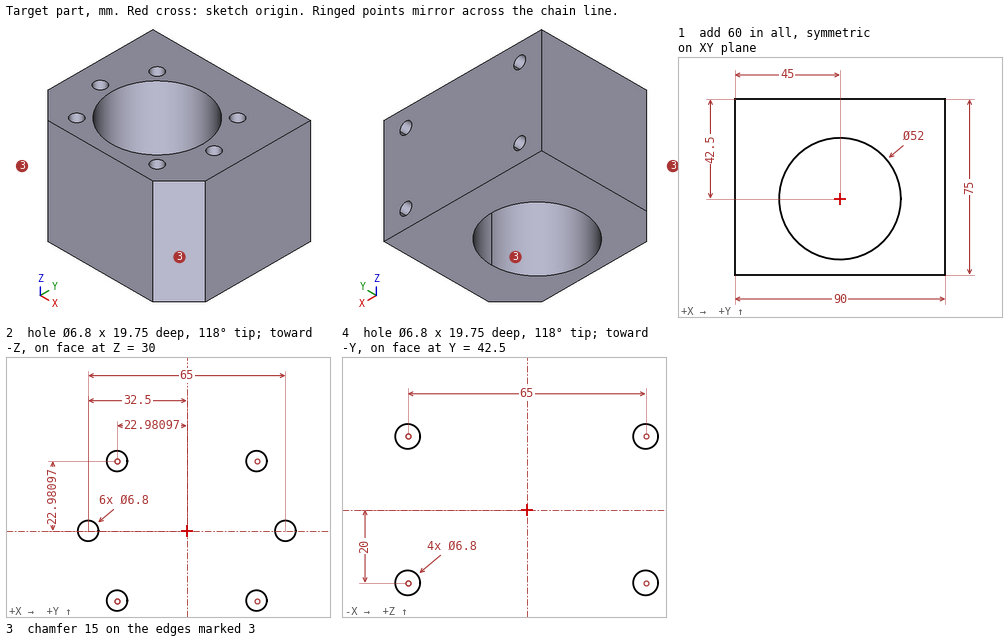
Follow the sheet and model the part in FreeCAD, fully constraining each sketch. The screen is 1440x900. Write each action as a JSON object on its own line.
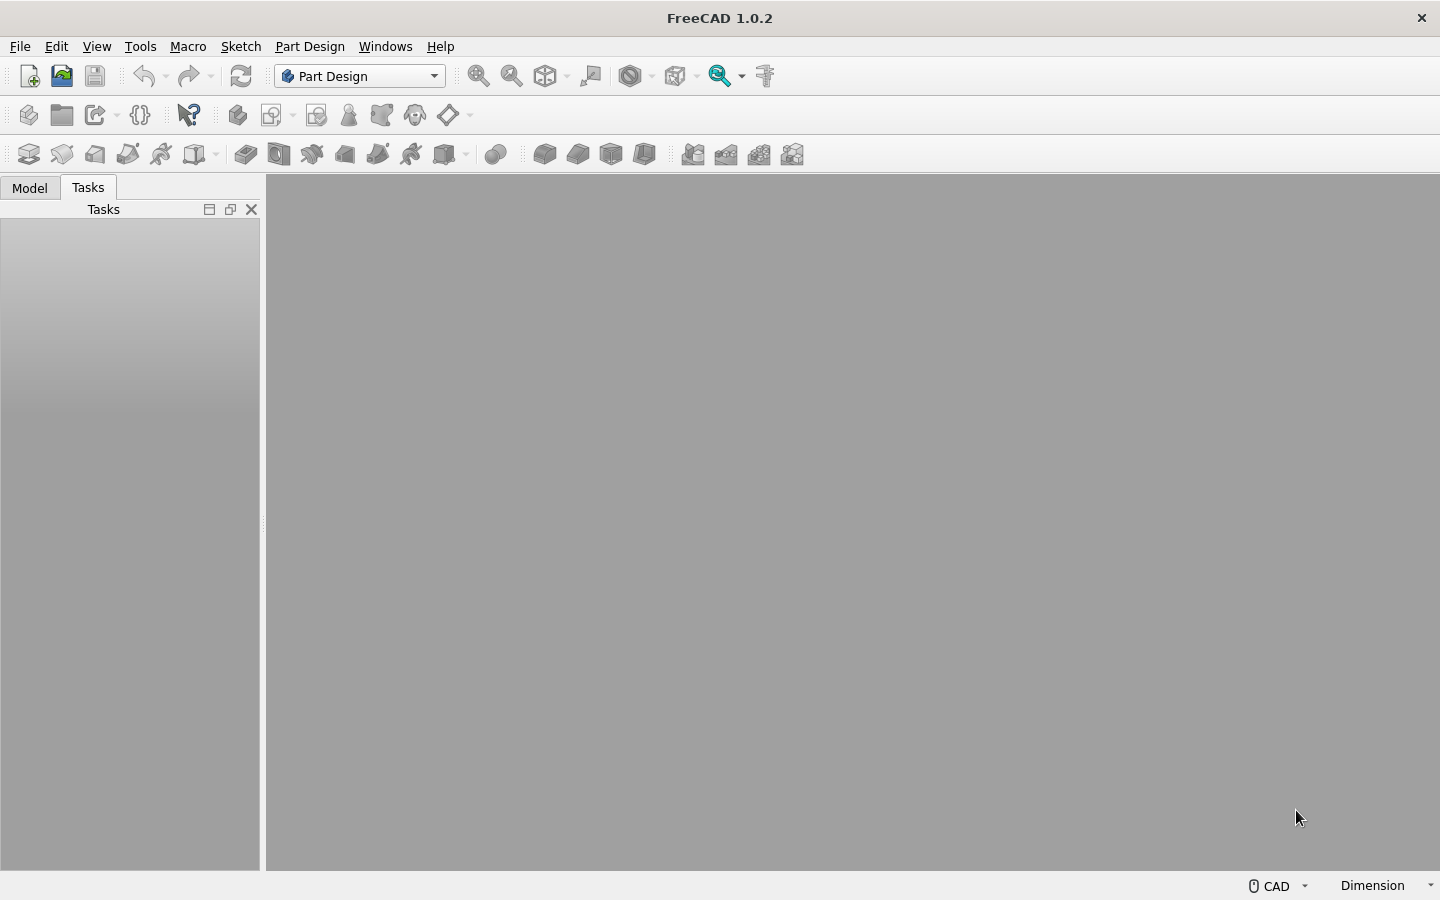
{"action": "left_click", "coordinate": [29, 76]}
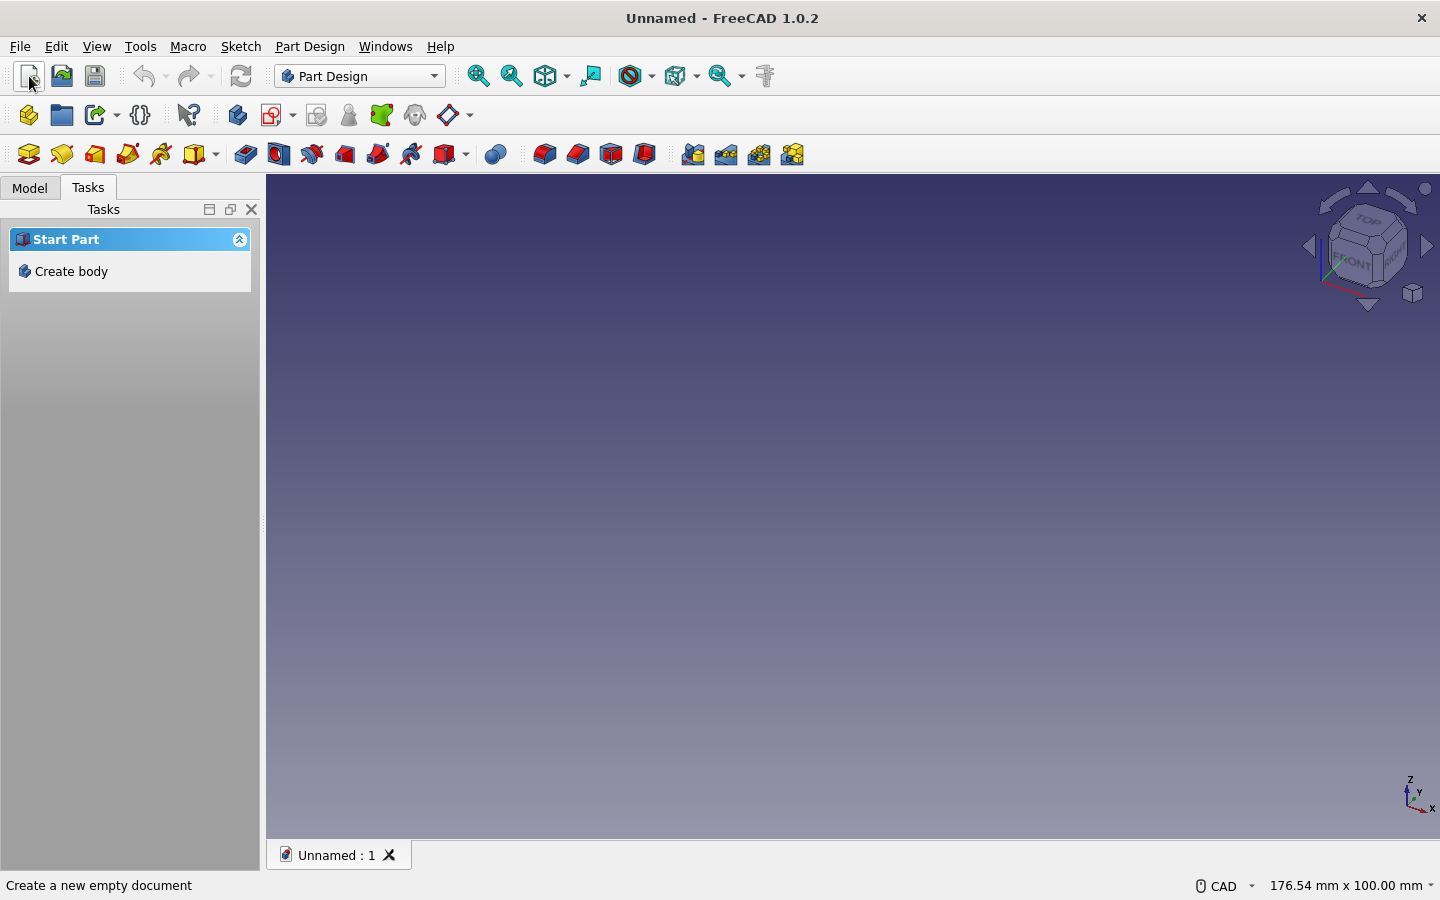
{"action": "left_click", "coordinate": [270, 116]}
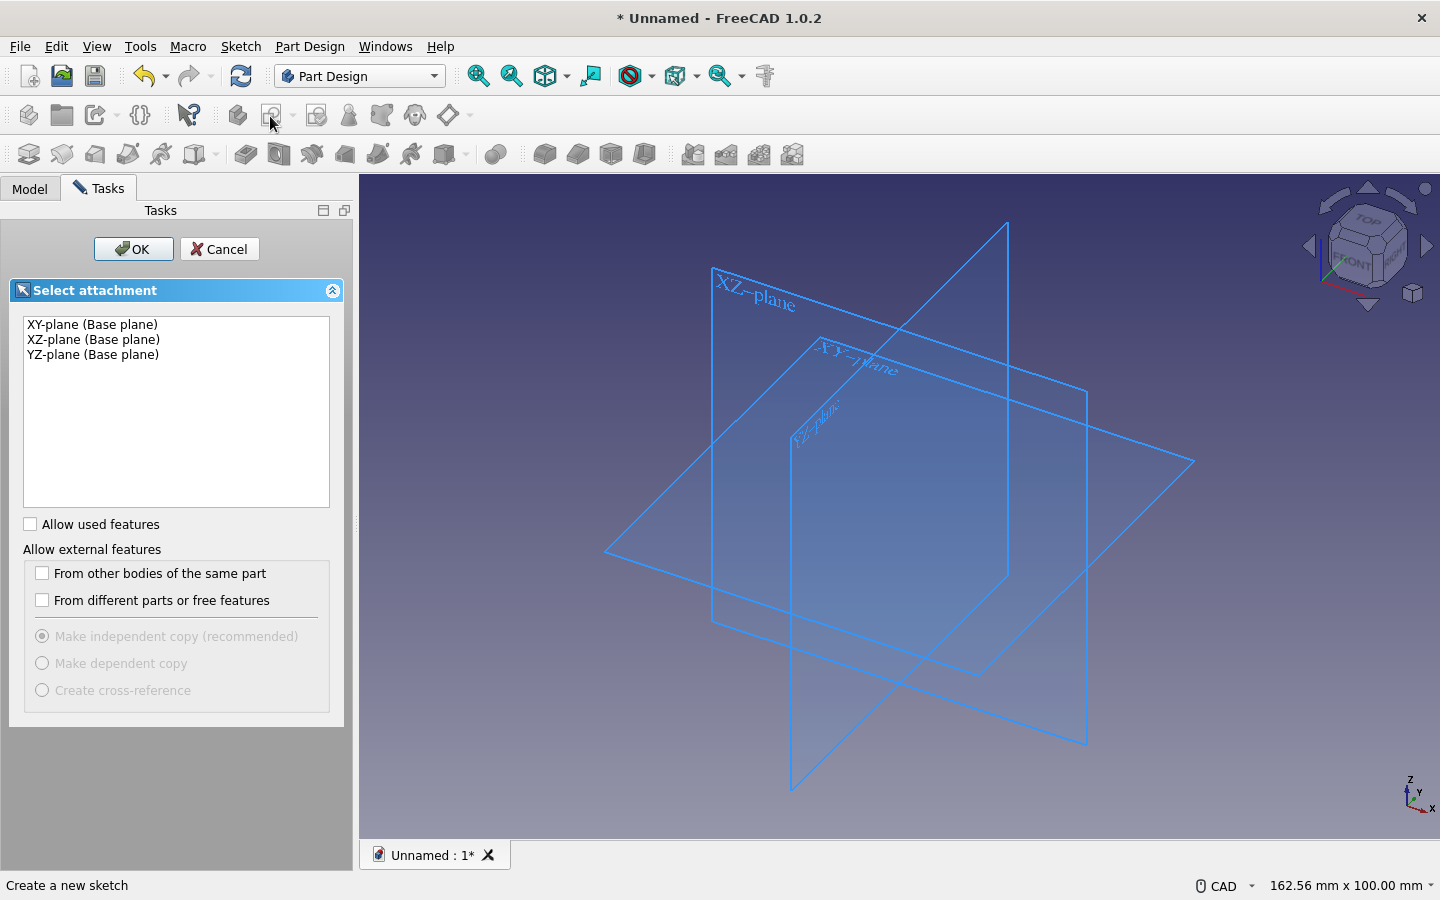
{"action": "left_click", "coordinate": [84, 324]}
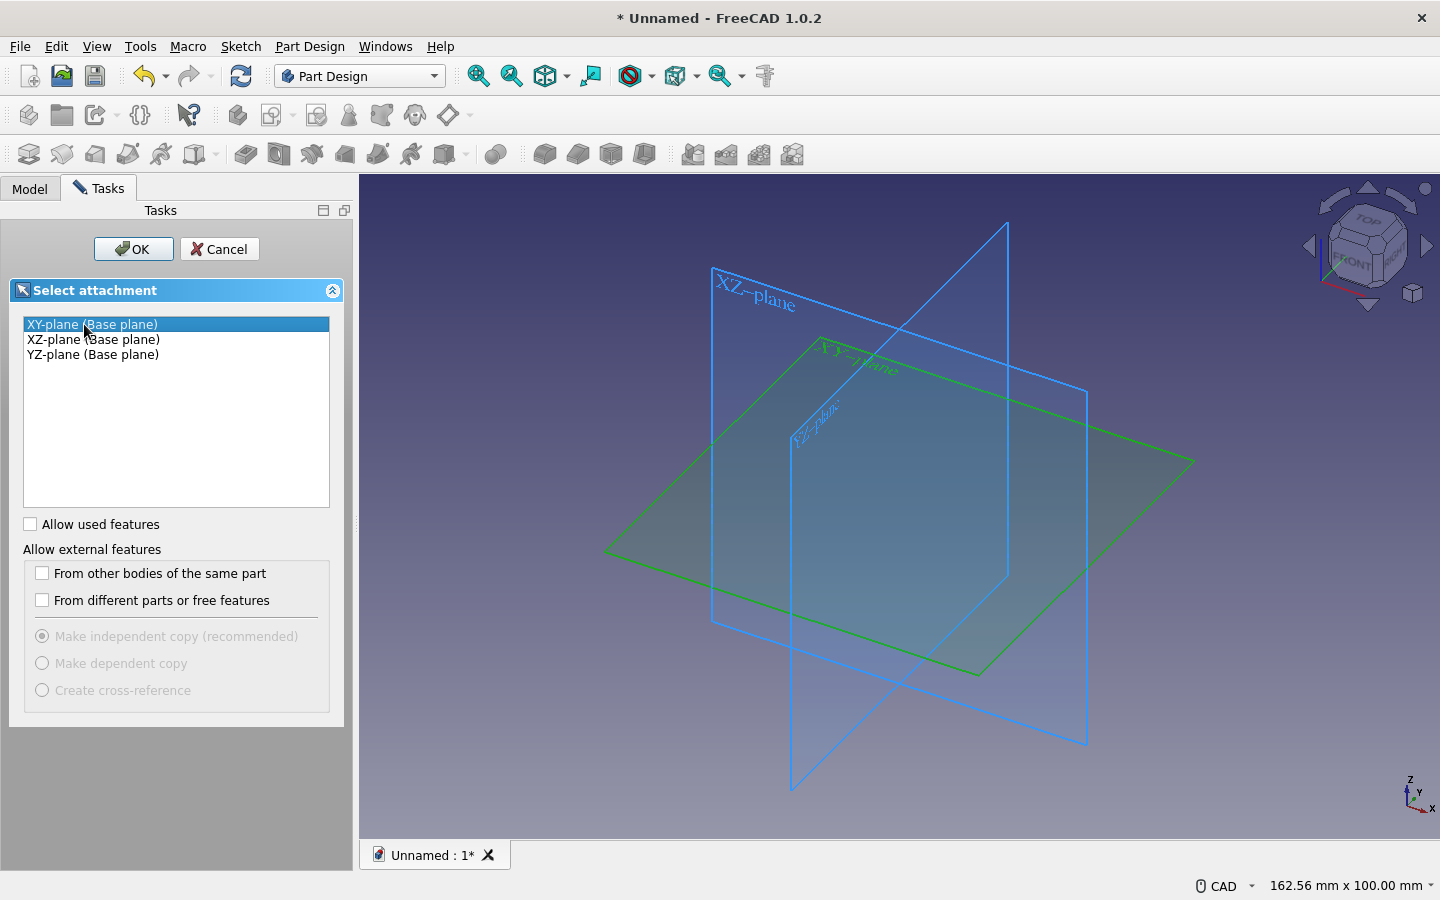
{"action": "left_click", "coordinate": [134, 249]}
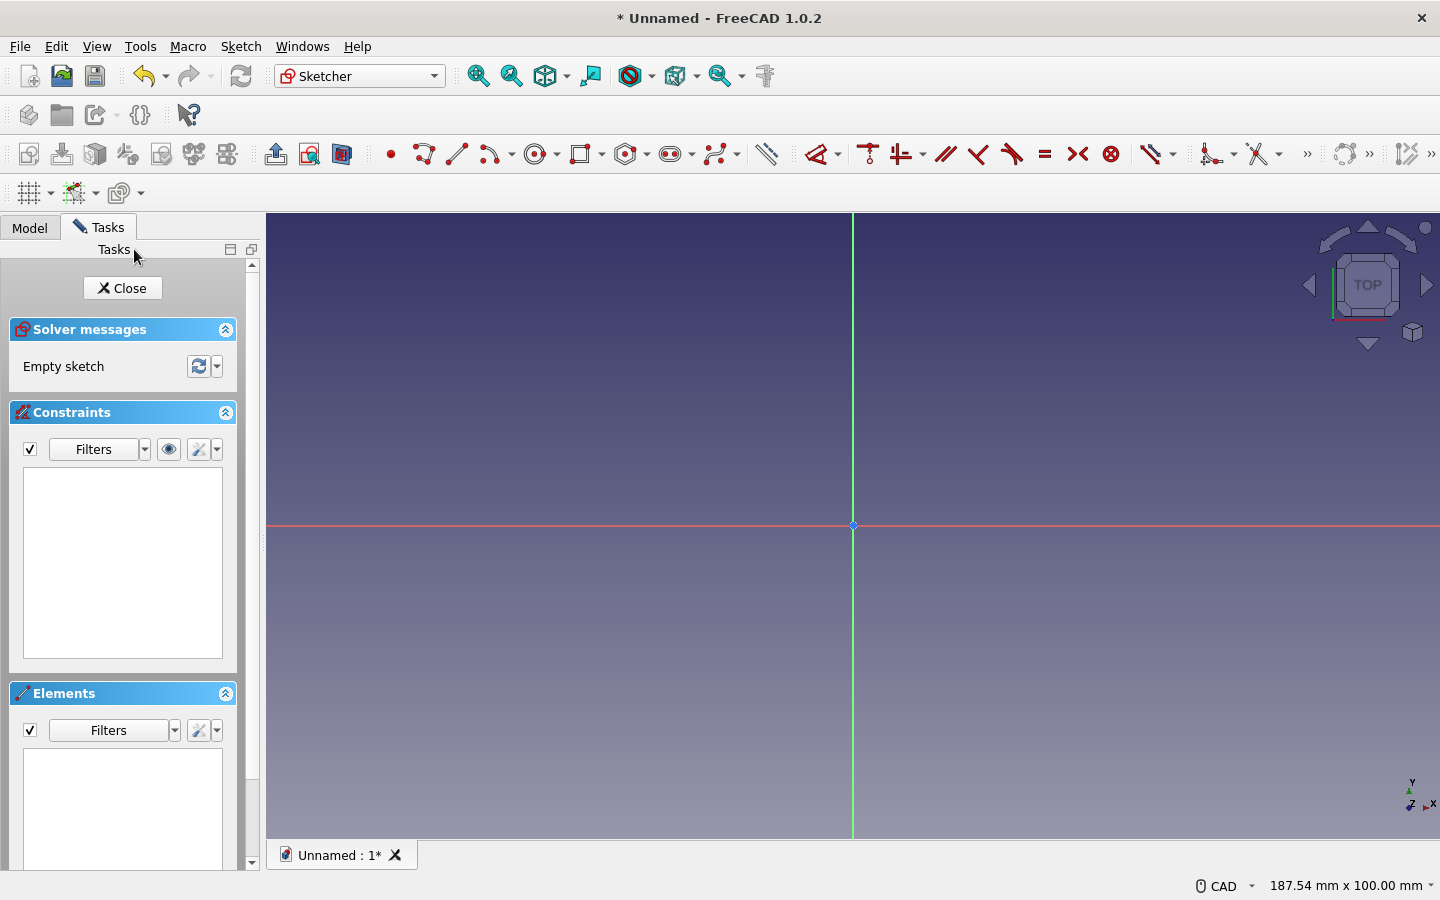
{"action": "scroll", "coordinate": [475, 667], "scroll_direction": "down", "scroll_amount": 1}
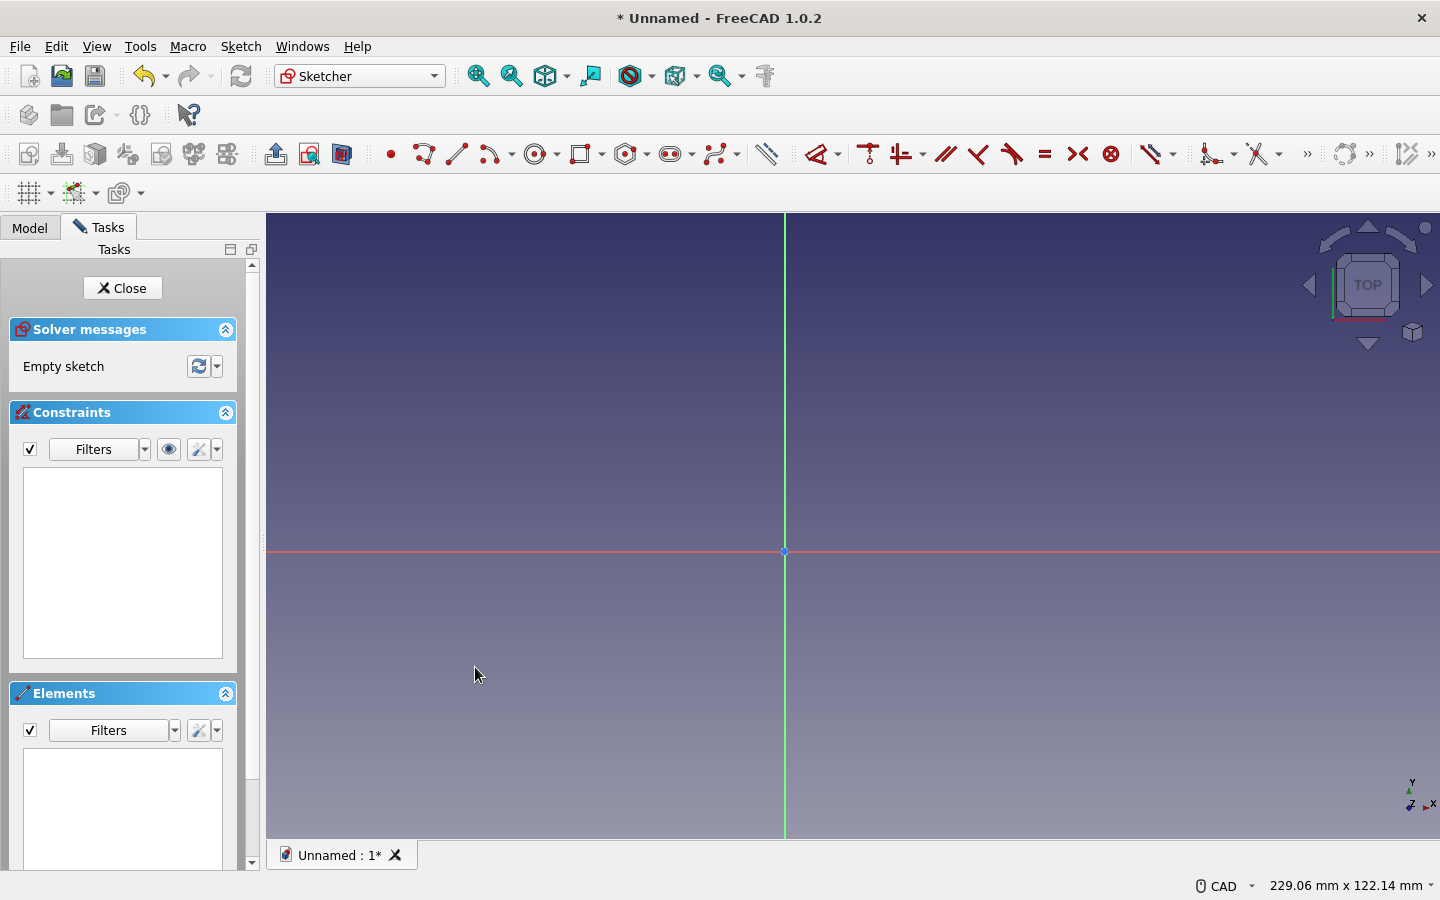
{"action": "left_click", "coordinate": [580, 154]}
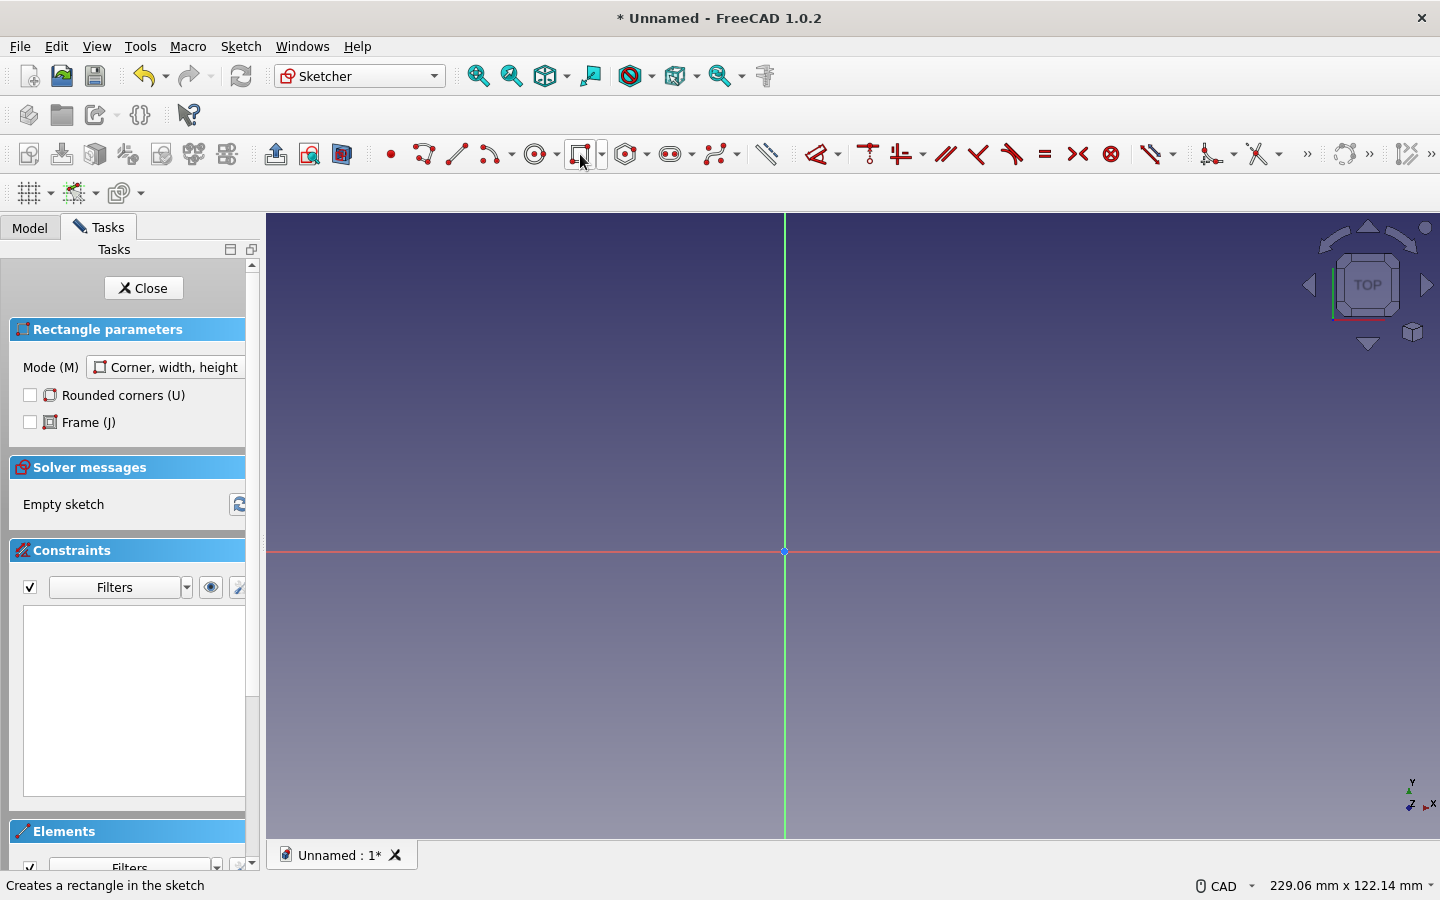
{"action": "left_click", "coordinate": [554, 334]}
{"action": "mouse_move", "coordinate": [1015, 718]}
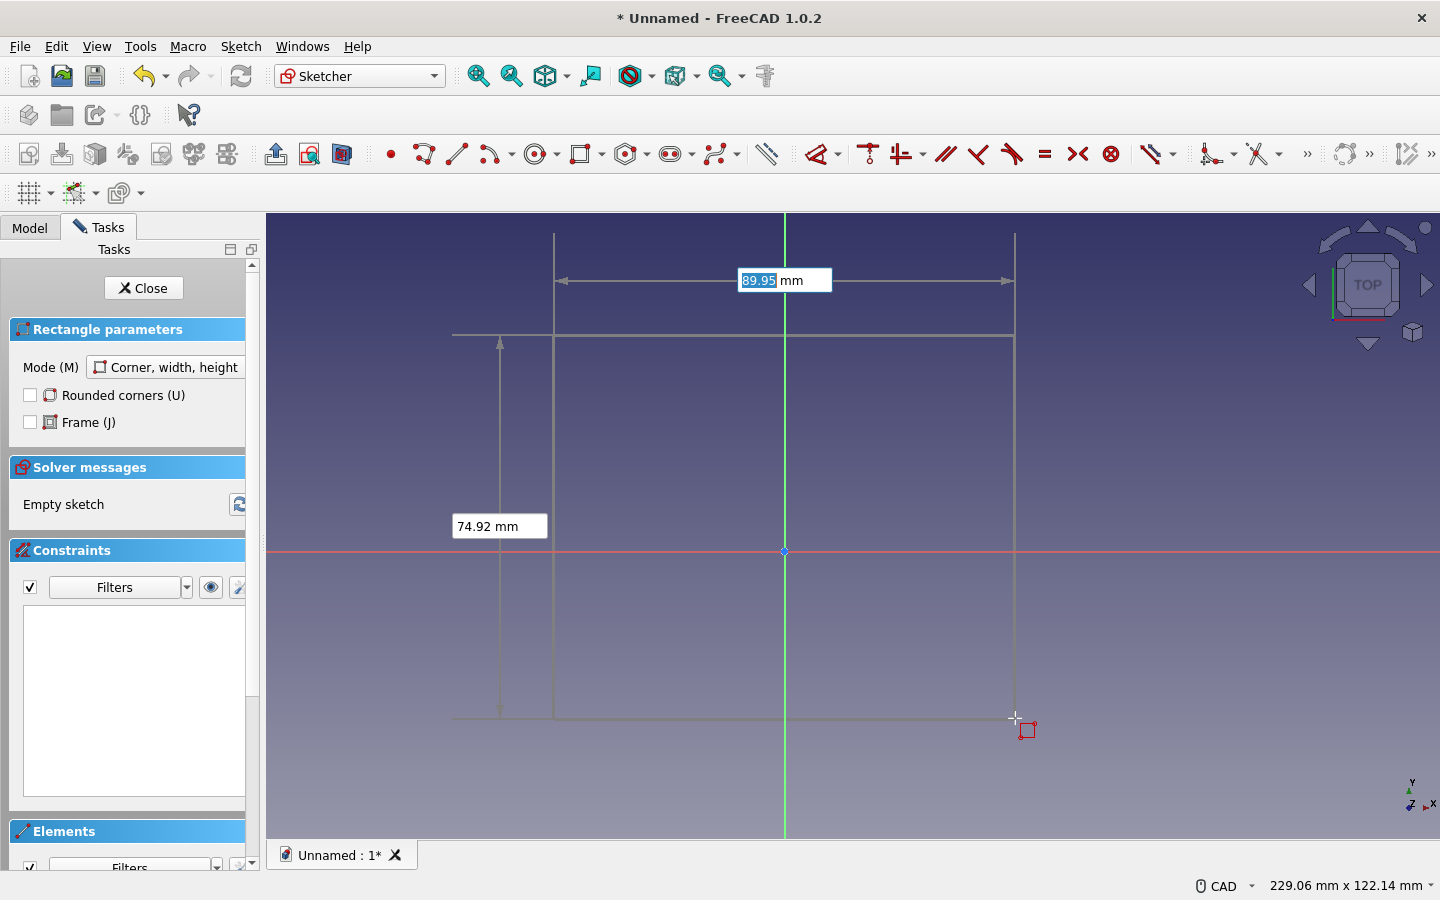
{"action": "type", "text": "90"}
{"action": "key", "text": "Tab"}
{"action": "type", "text": "75"}
{"action": "key", "text": "Return"}